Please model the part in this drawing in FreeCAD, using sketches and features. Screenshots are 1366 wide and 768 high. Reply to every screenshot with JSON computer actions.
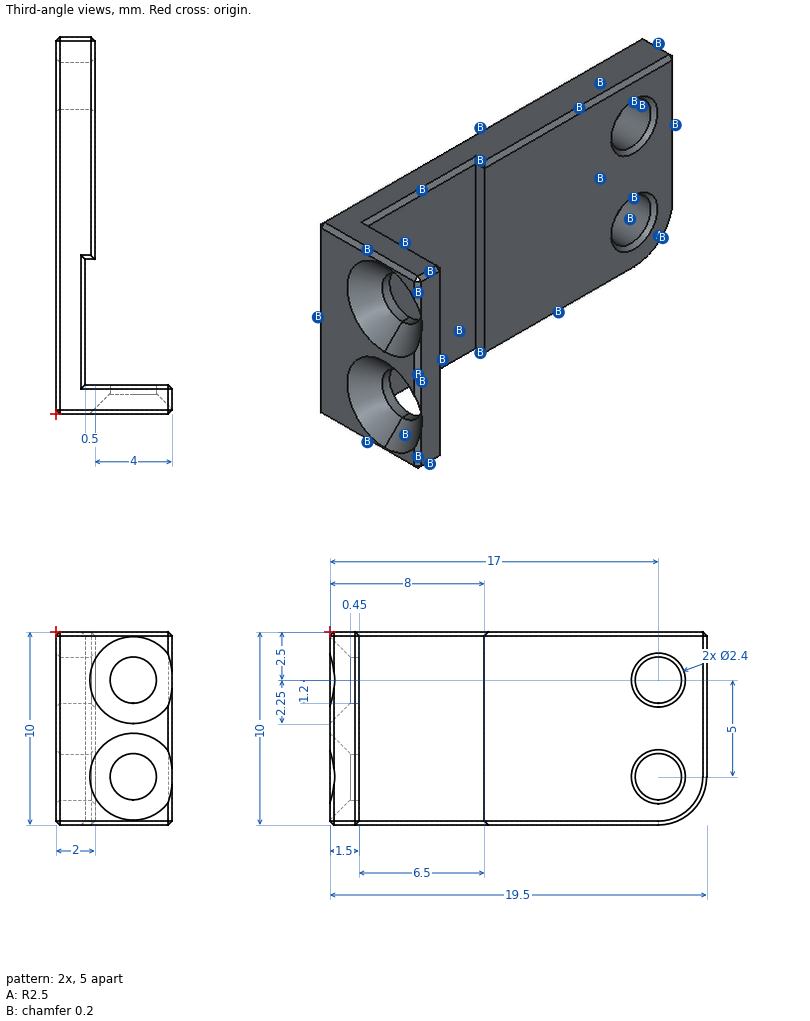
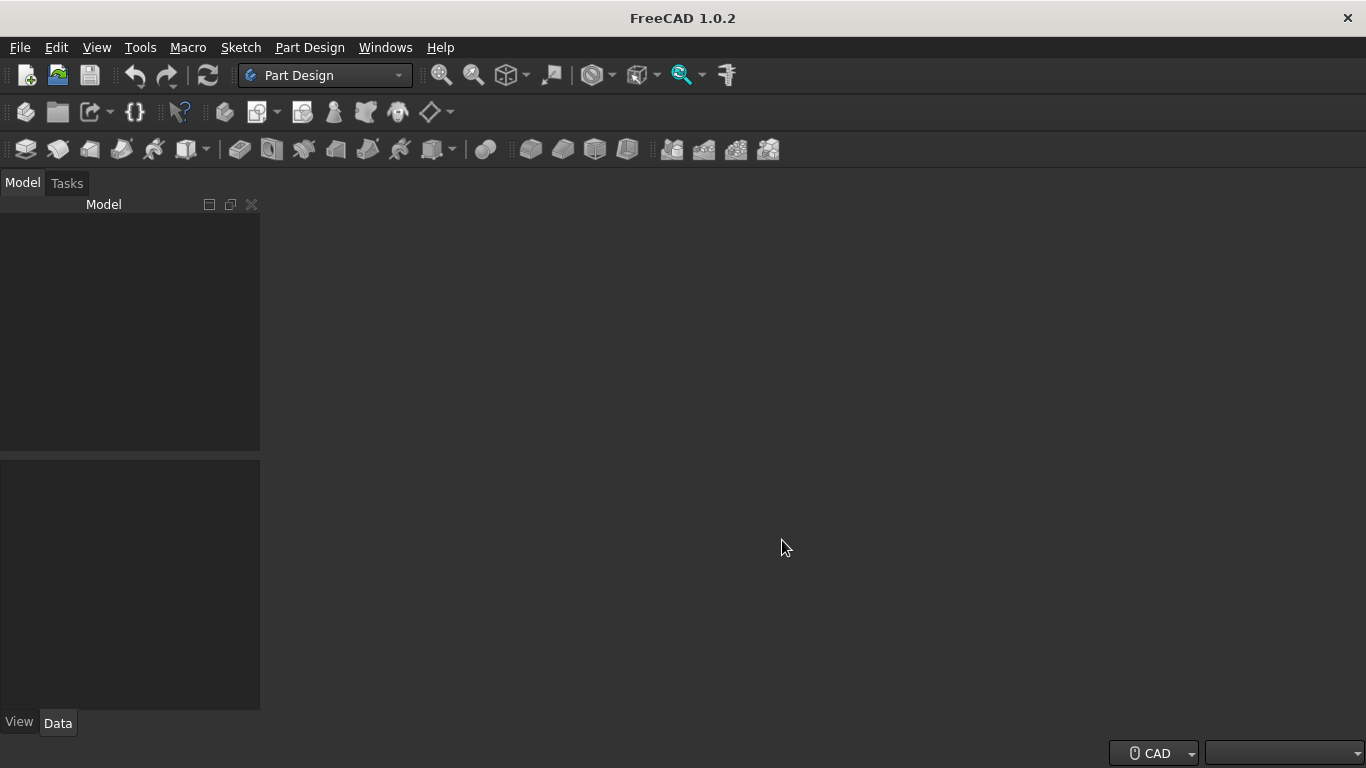
{"action": "left_click", "coordinate": [26, 76]}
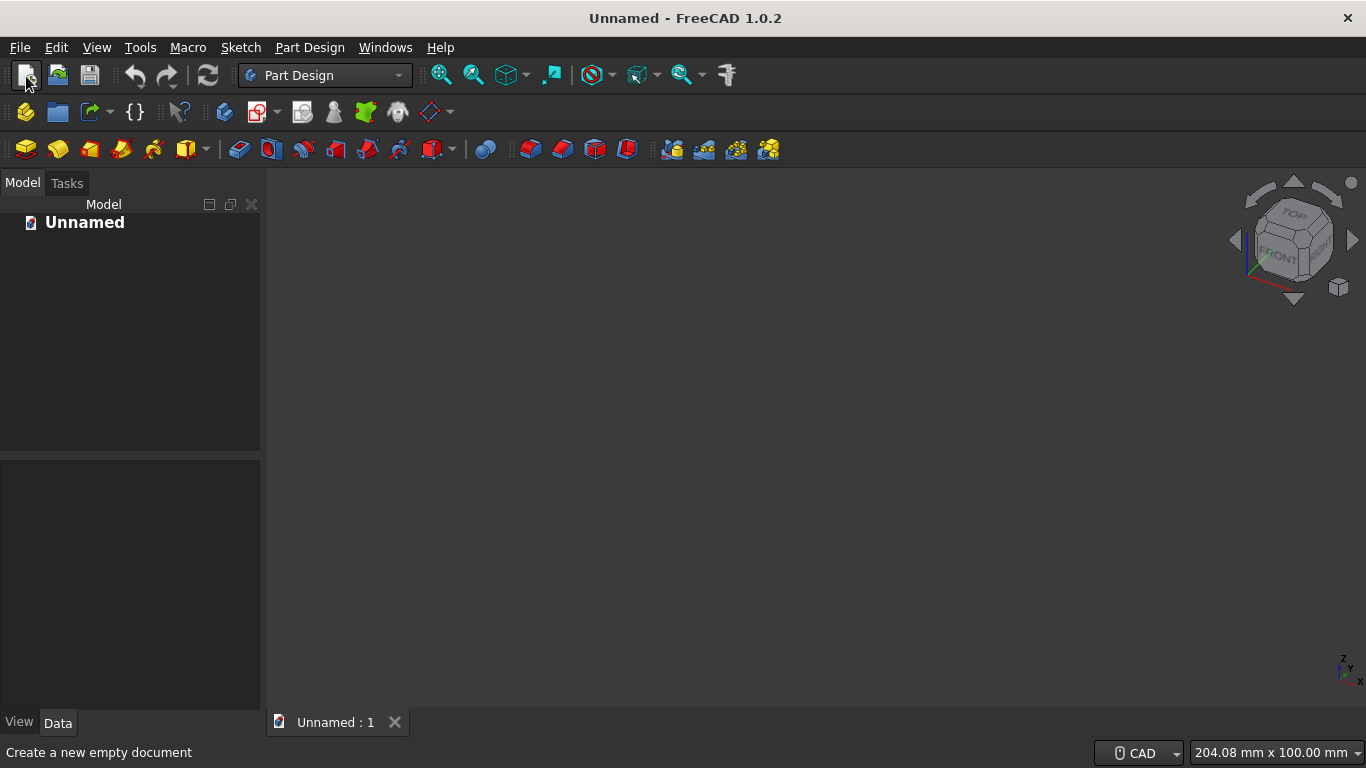
{"action": "left_click", "coordinate": [258, 112]}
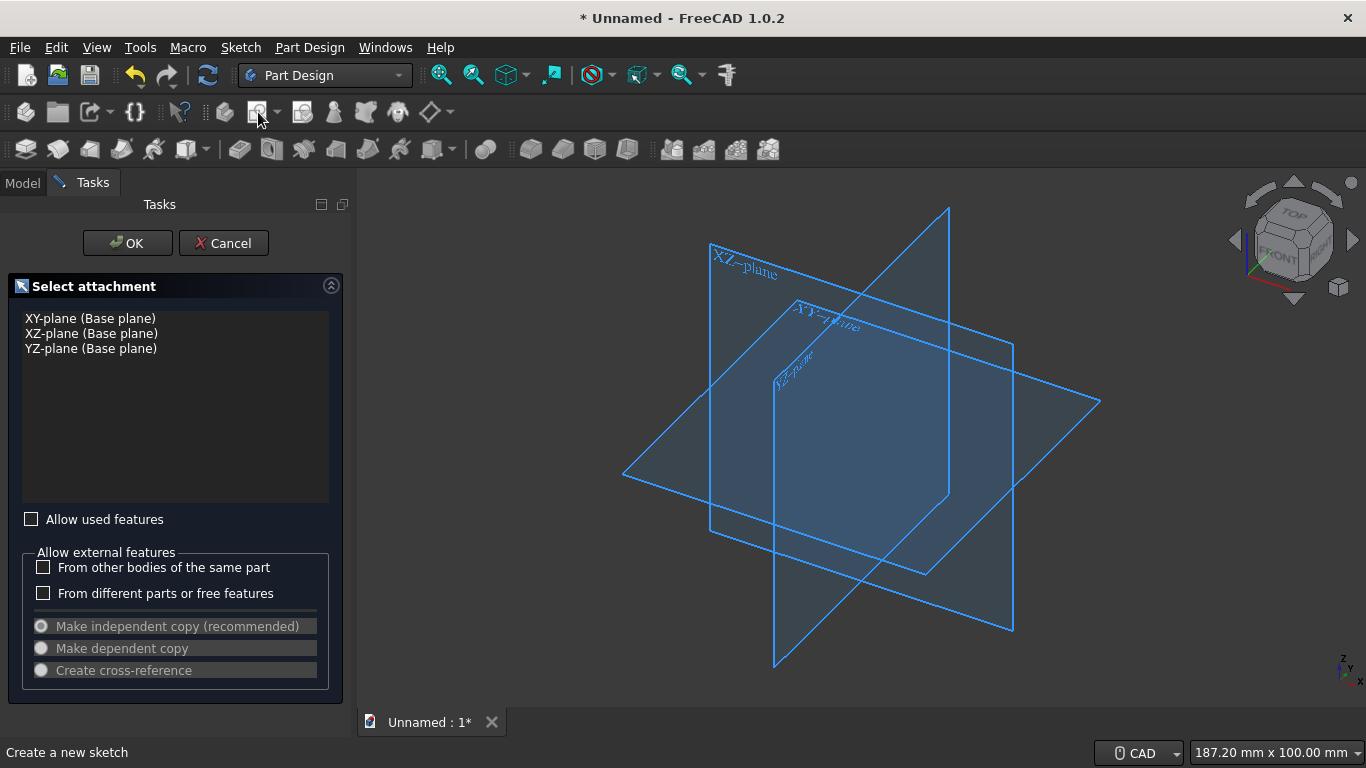
{"action": "left_click", "coordinate": [82, 334]}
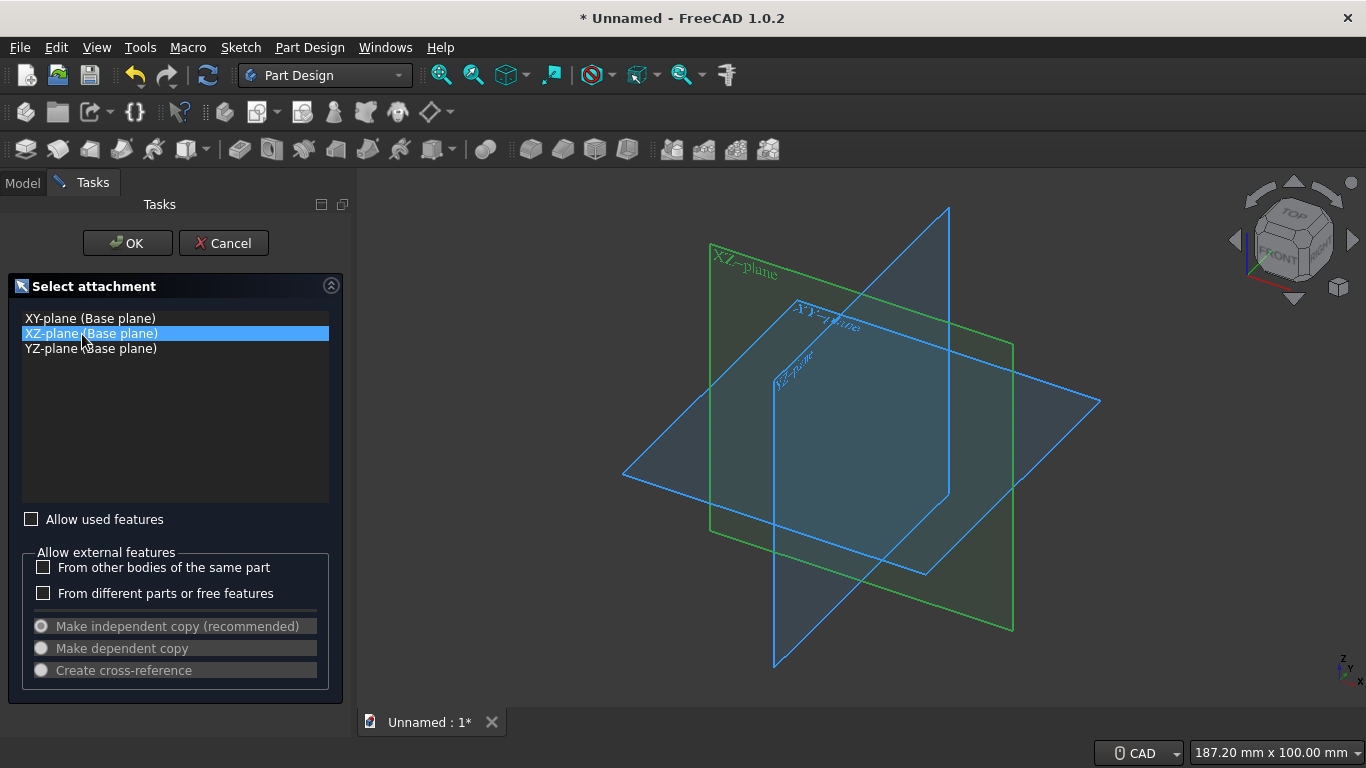
{"action": "left_click", "coordinate": [128, 243]}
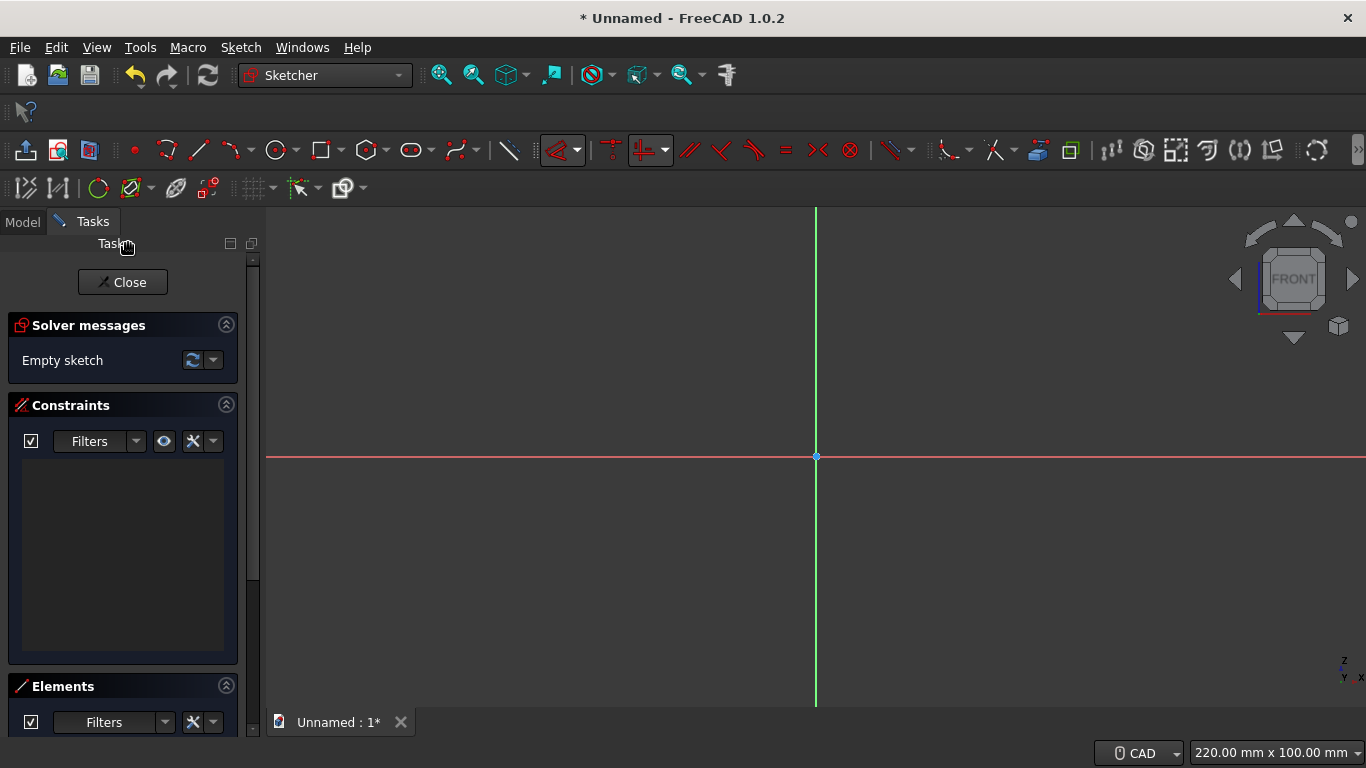
{"action": "scroll", "coordinate": [836, 487], "scroll_direction": "up", "scroll_amount": 9}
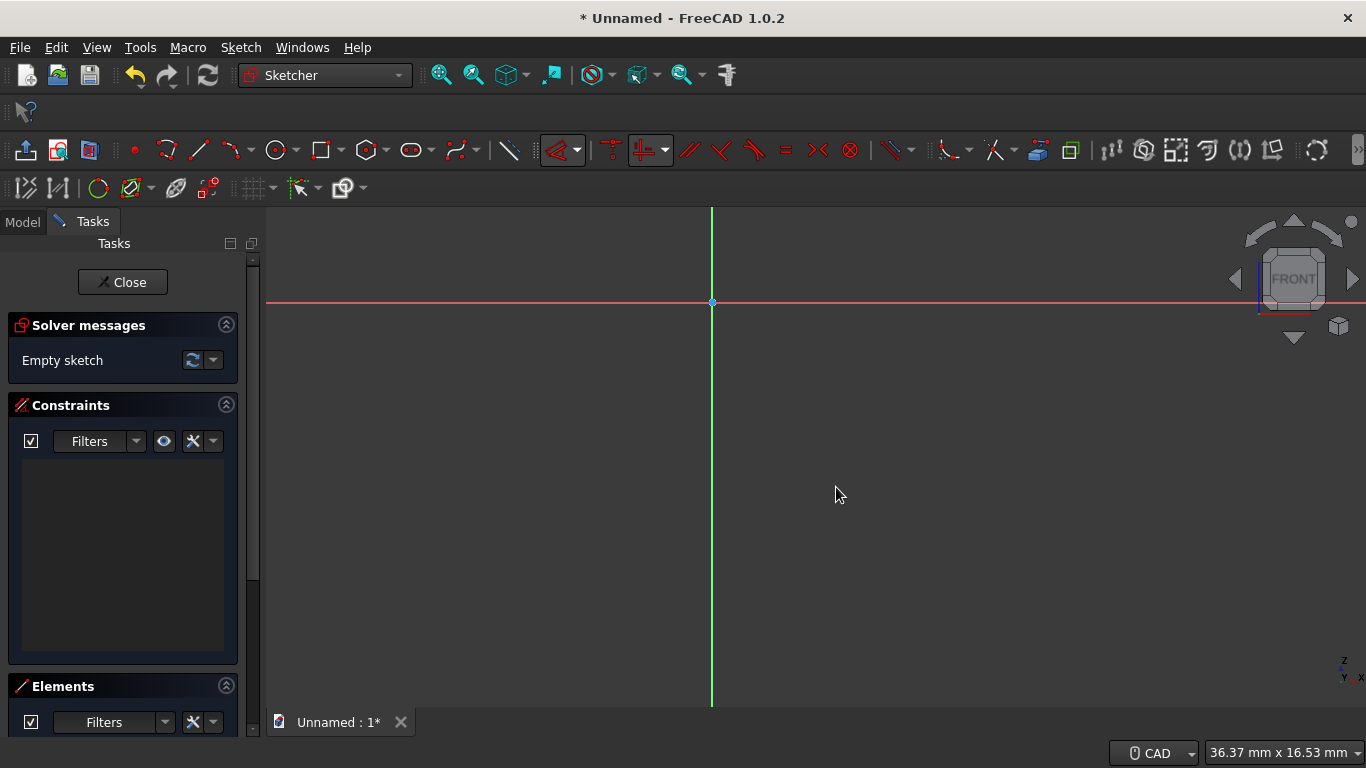
{"action": "left_click", "coordinate": [322, 150]}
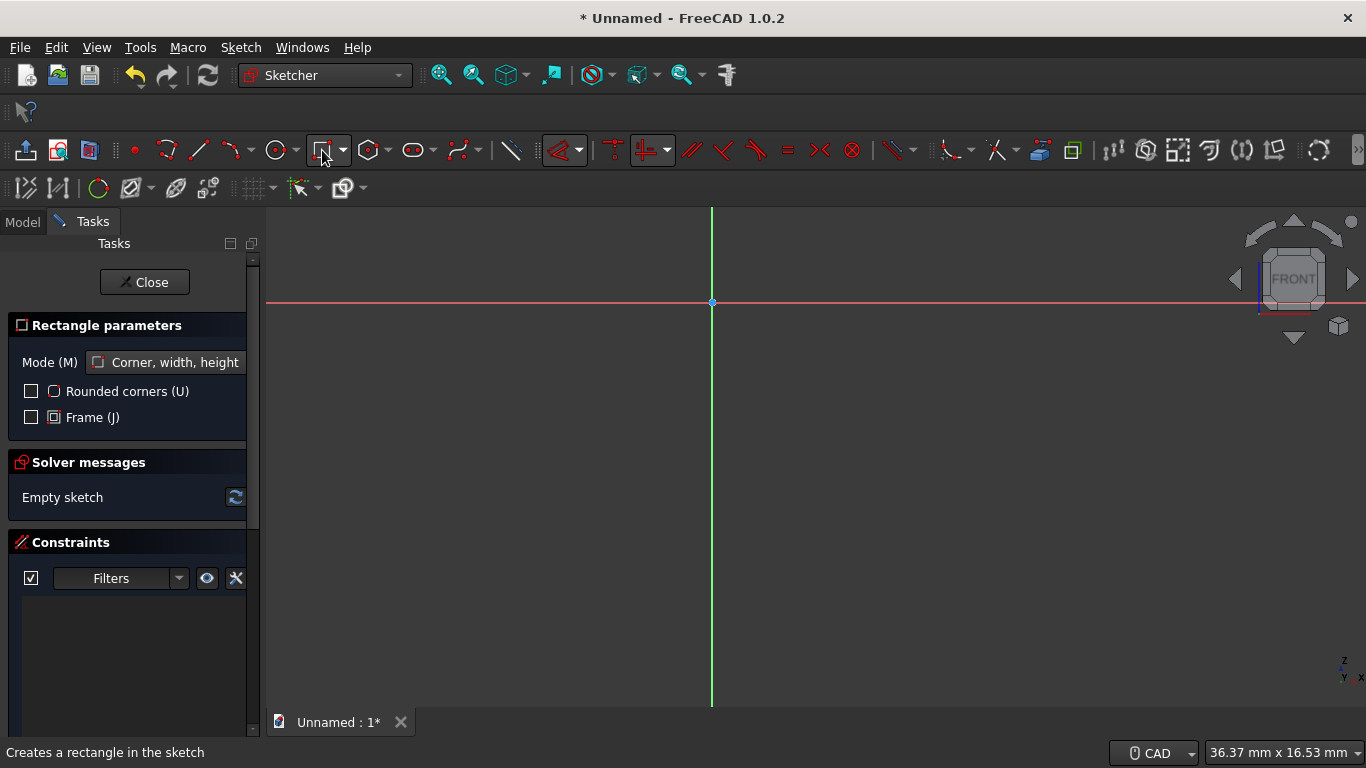
{"action": "left_click", "coordinate": [712, 303]}
{"action": "left_click", "coordinate": [773, 605]}
{"action": "key", "text": "Escape"}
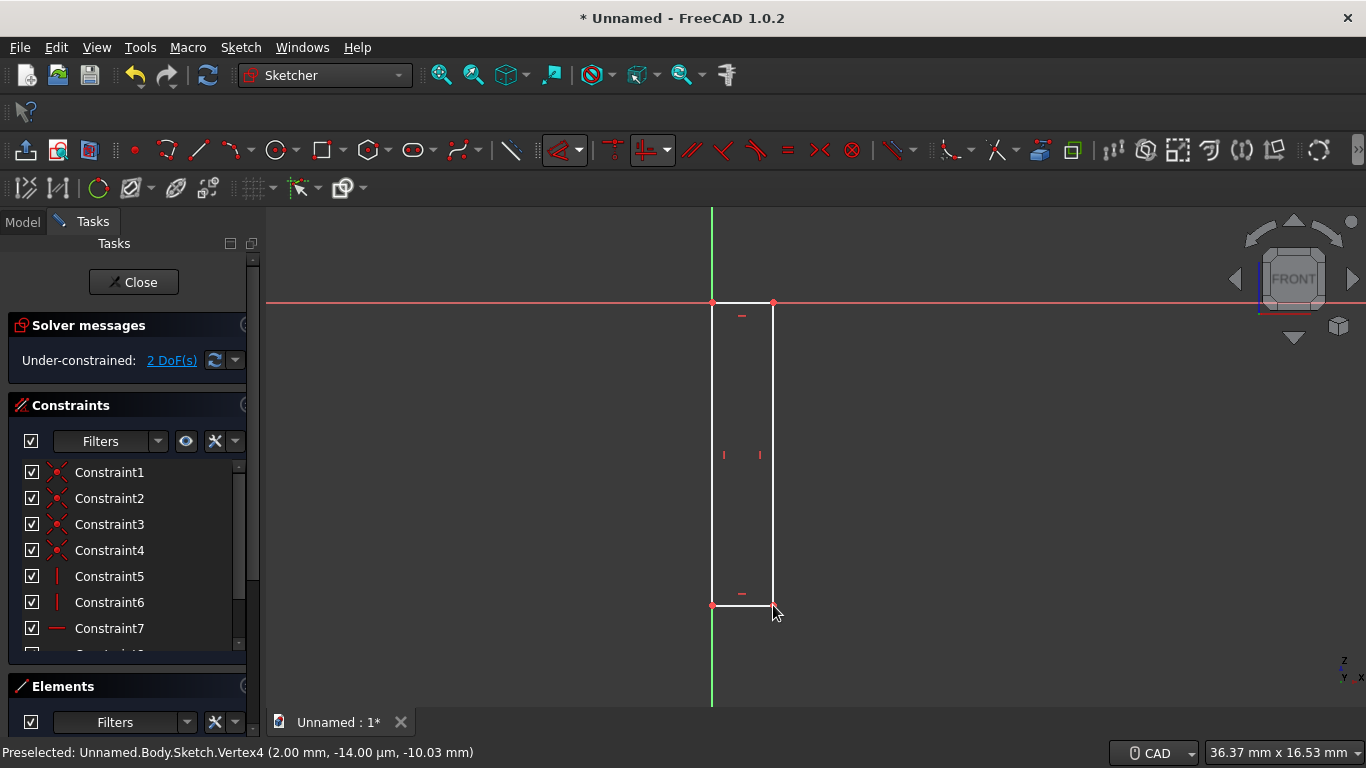
{"action": "left_click", "coordinate": [558, 150]}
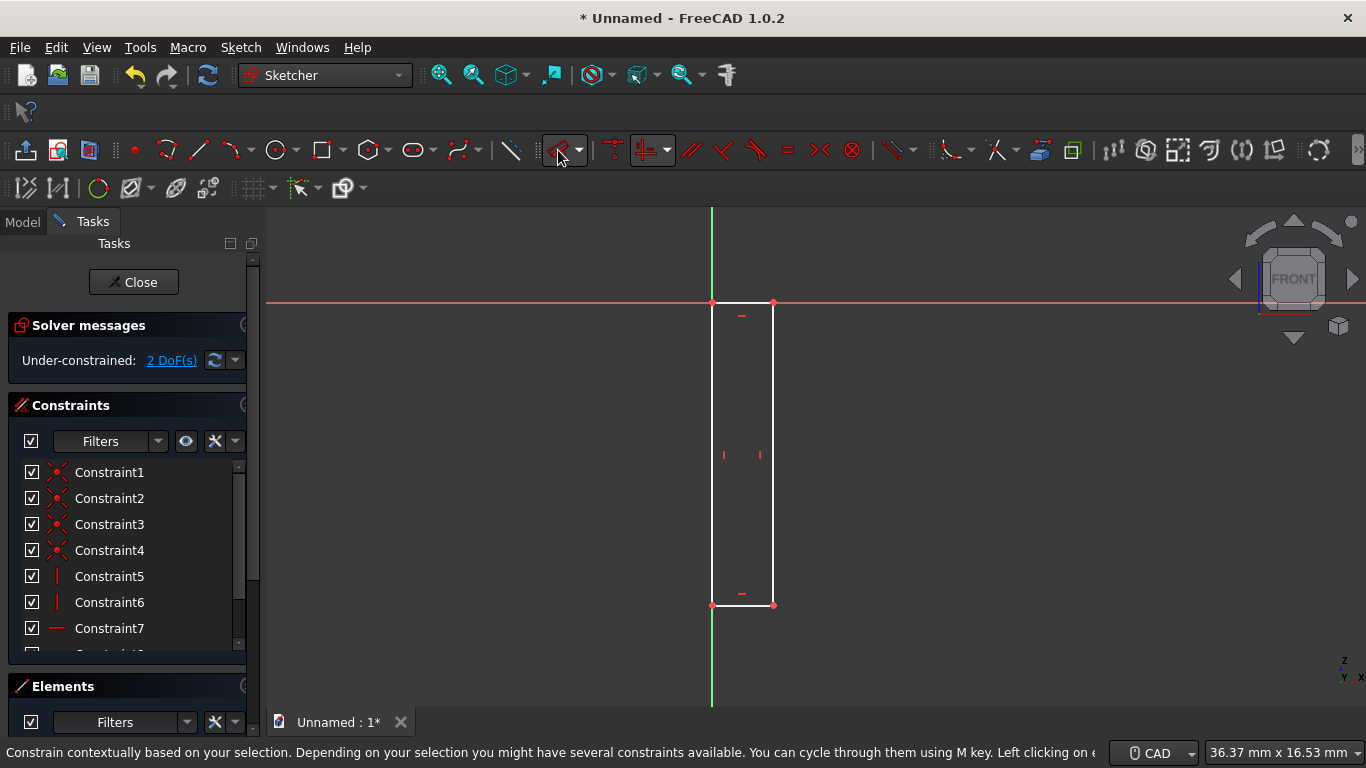
{"action": "left_click", "coordinate": [731, 606]}
{"action": "left_click", "coordinate": [743, 640]}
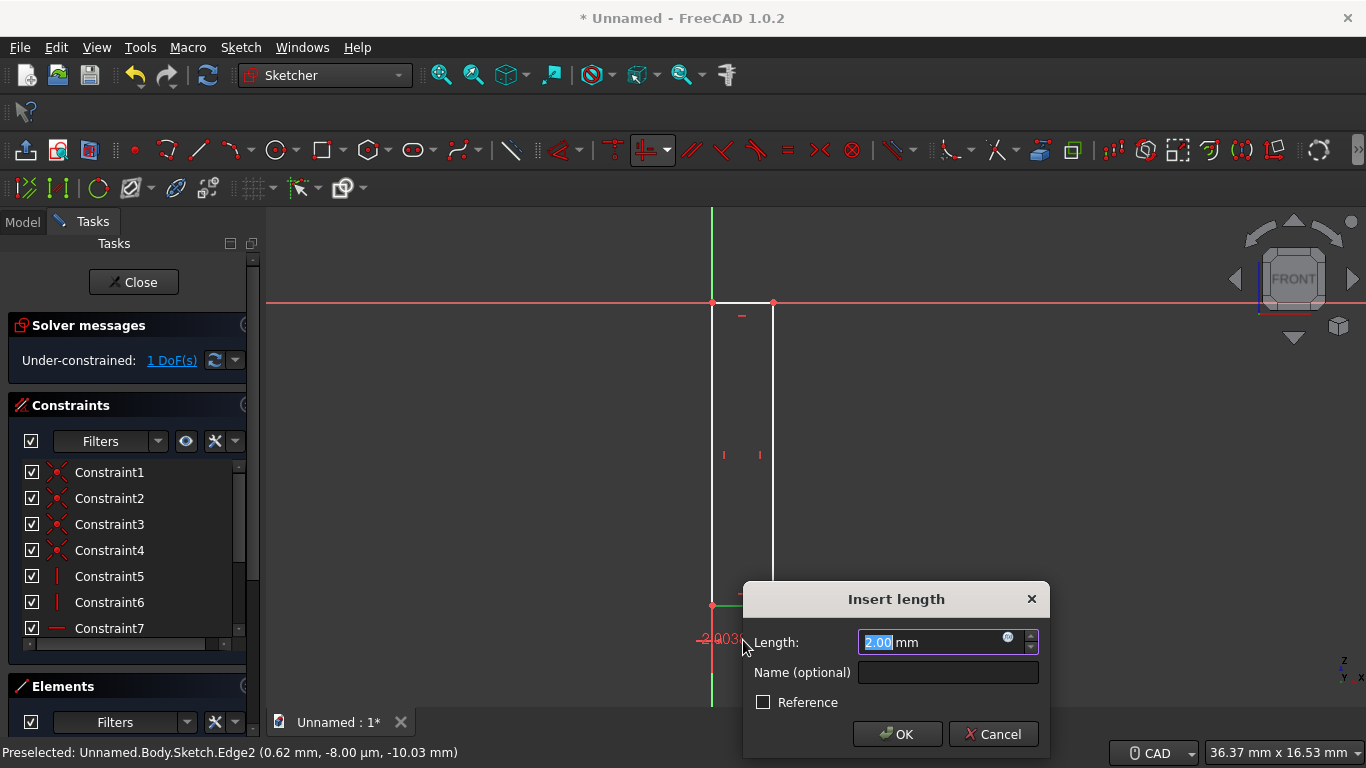
{"action": "type", "text": "2"}
{"action": "key", "text": "Return"}